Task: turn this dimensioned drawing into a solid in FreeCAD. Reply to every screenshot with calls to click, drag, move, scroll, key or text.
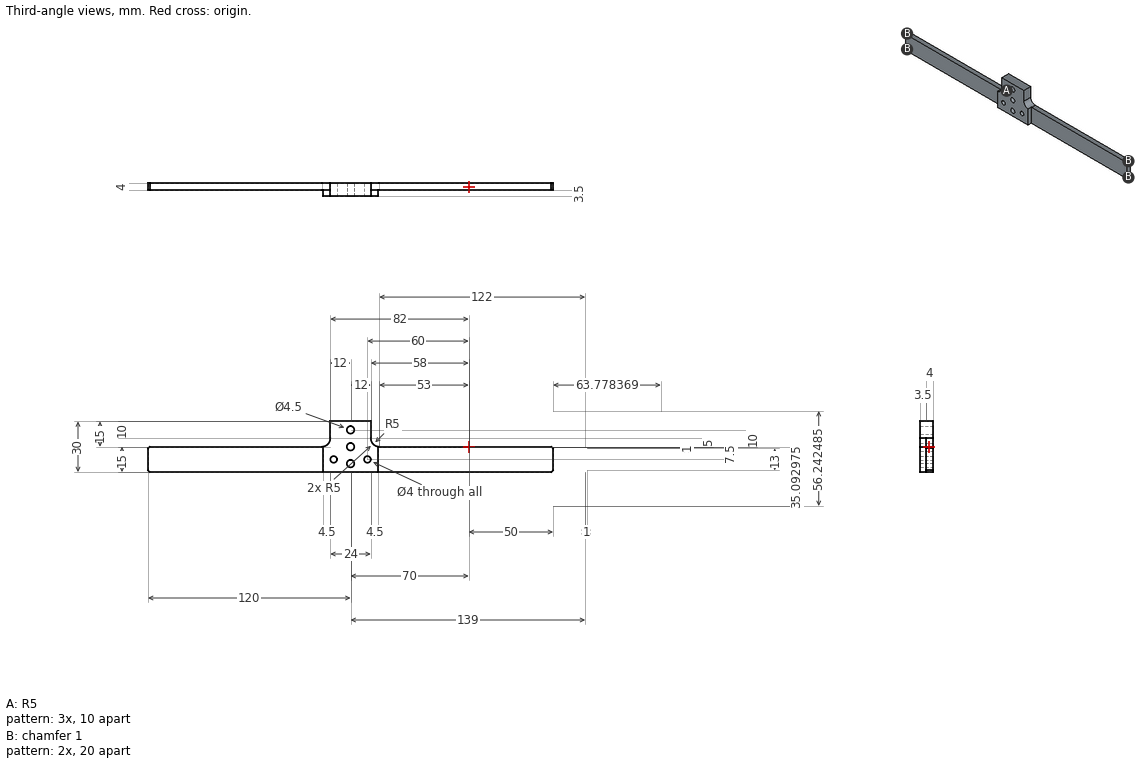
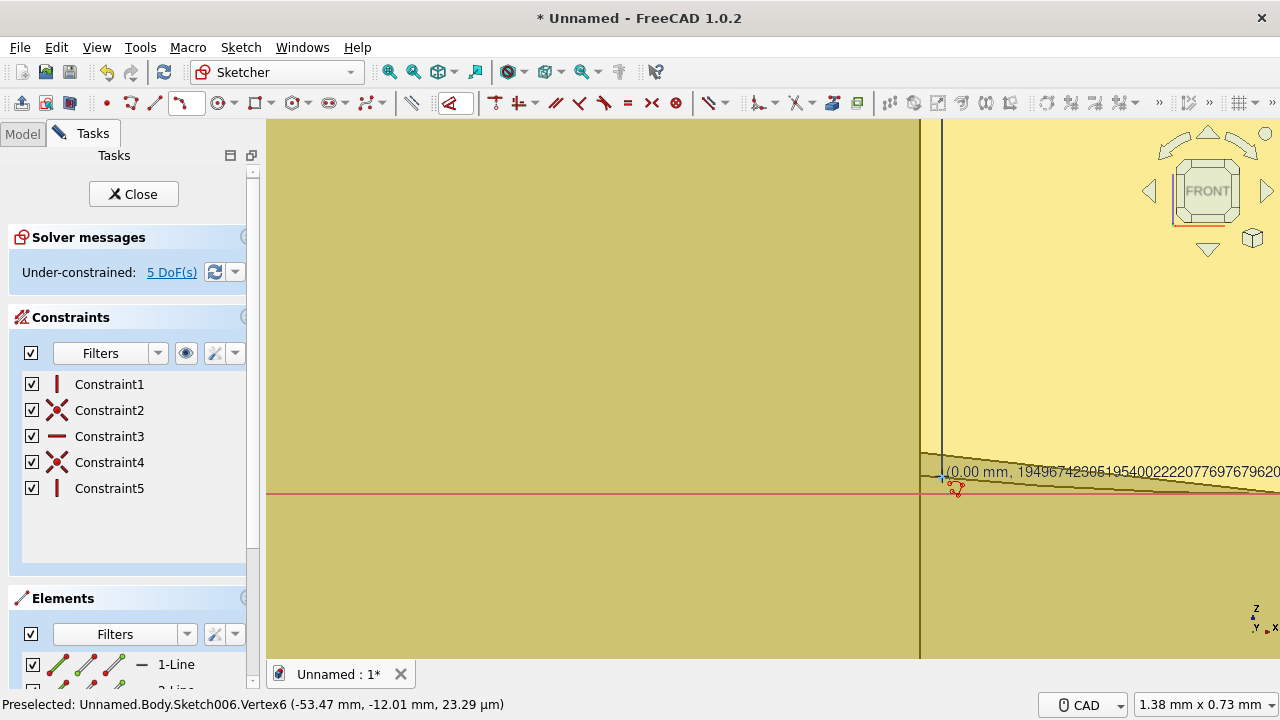
click(180, 104)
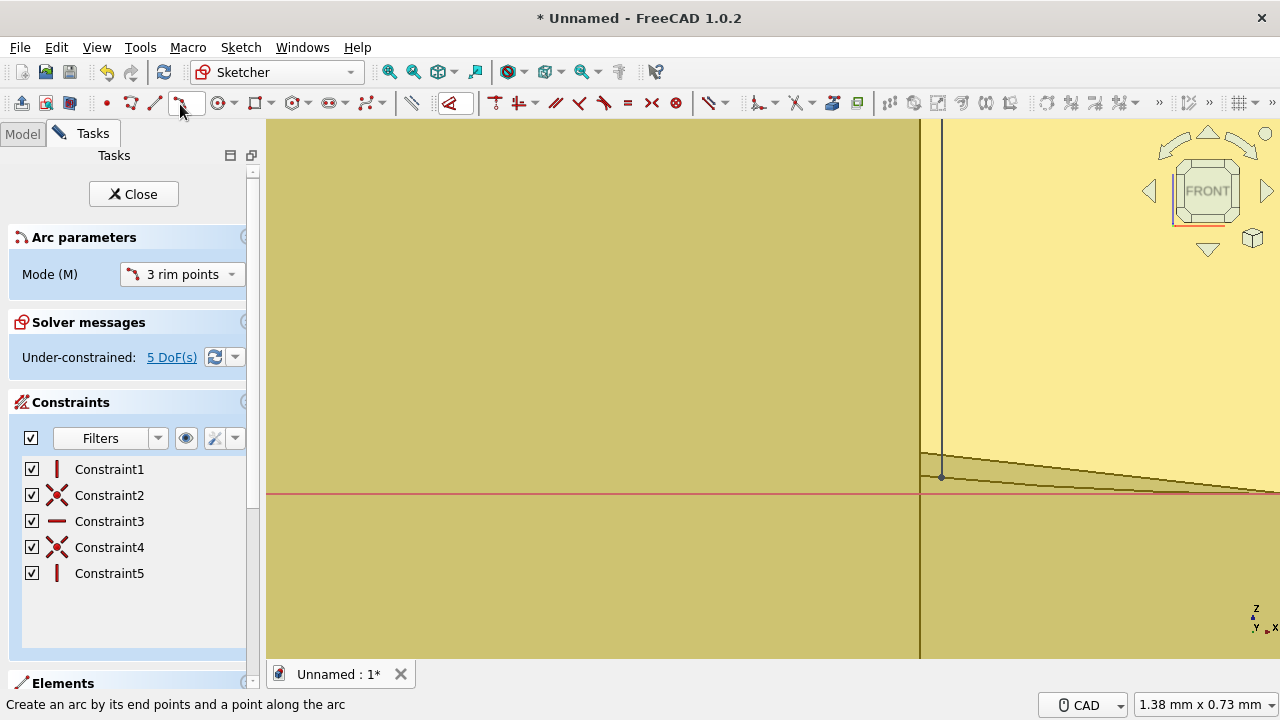
click(942, 477)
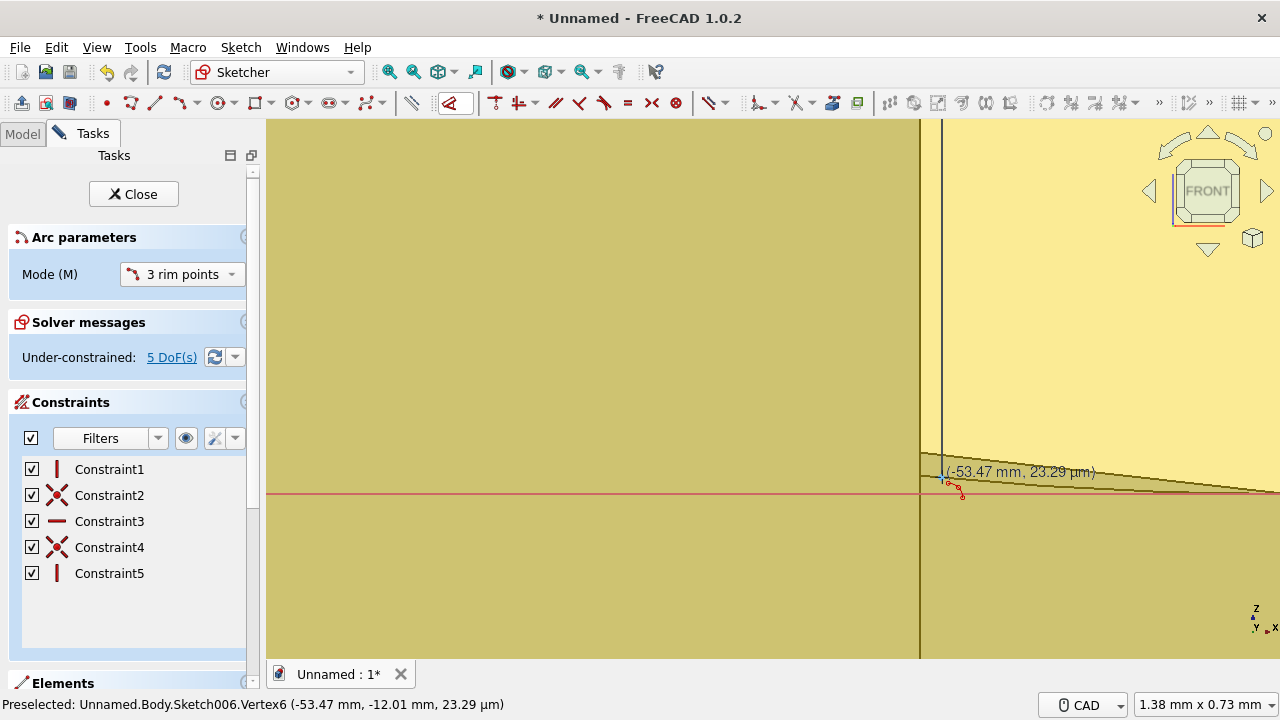
scroll(1040, 542, down, 18)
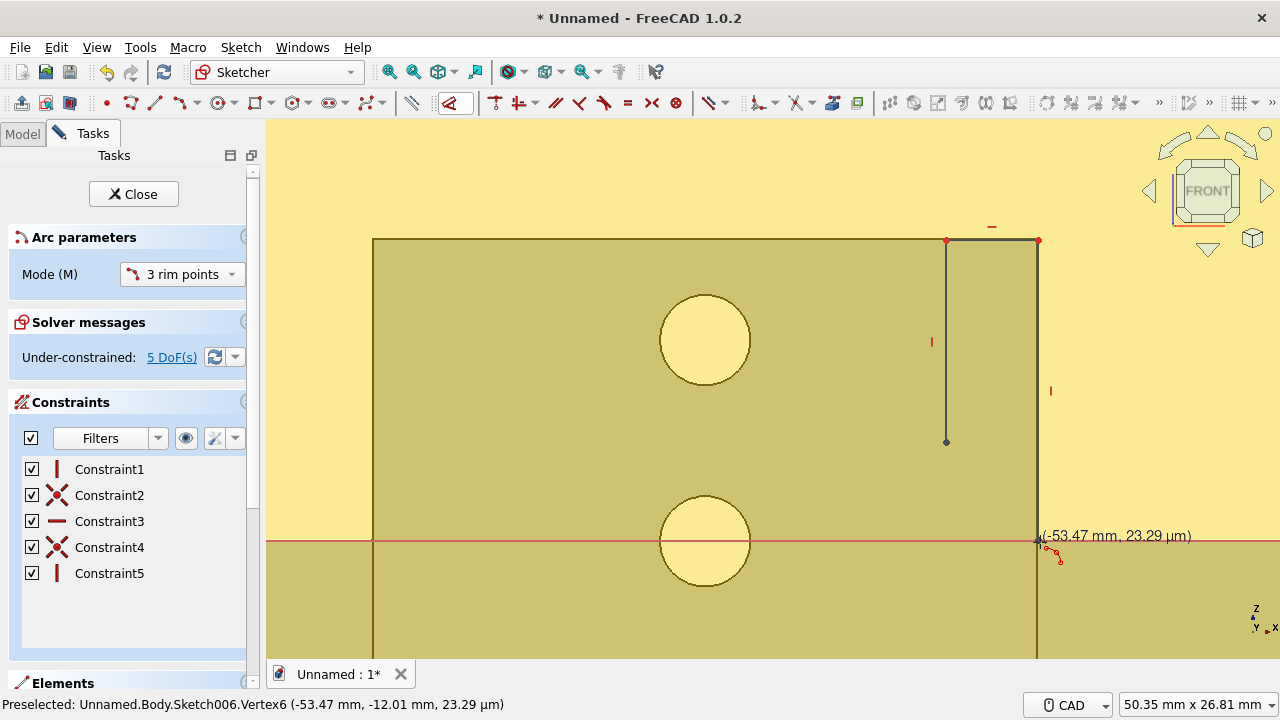
click(946, 442)
click(973, 508)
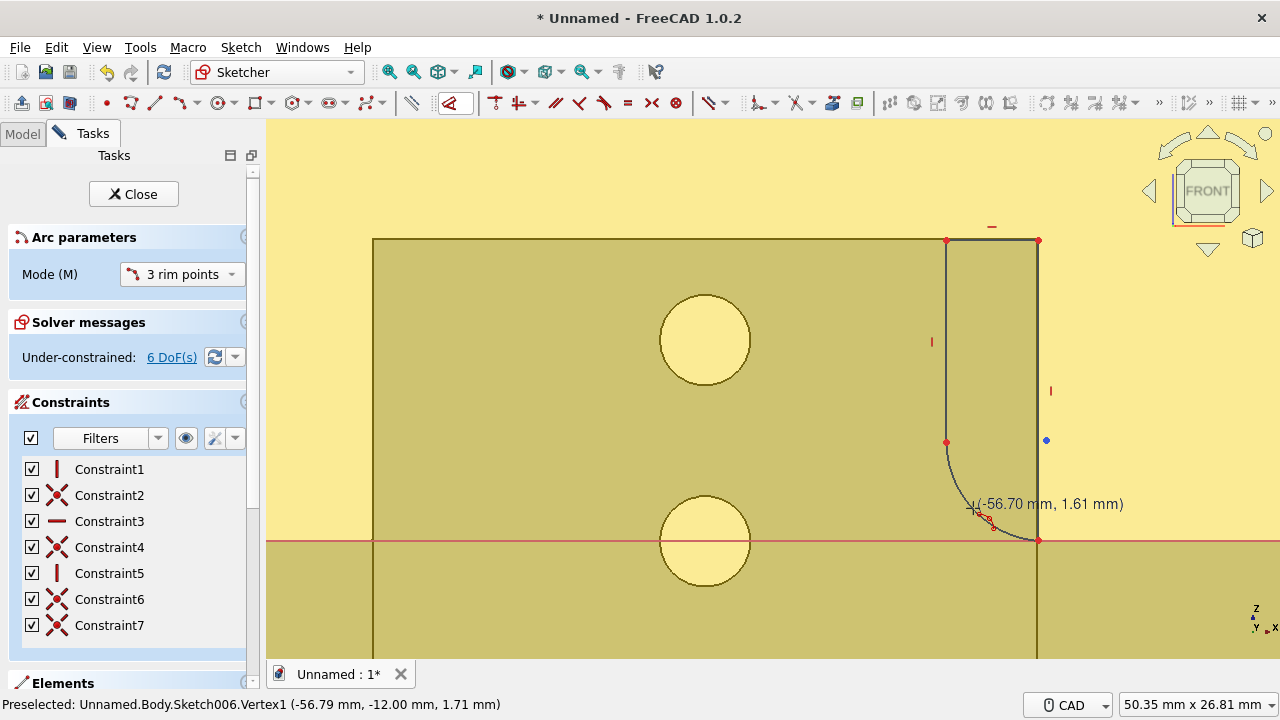
click(132, 104)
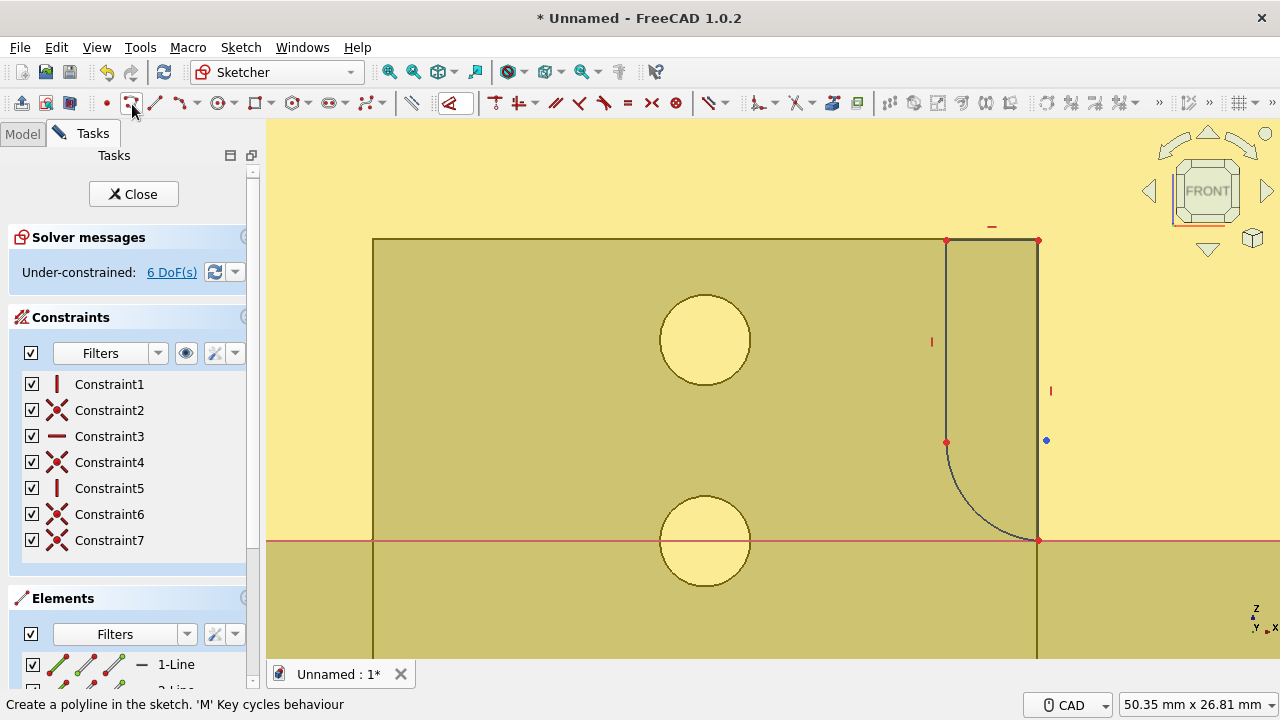
scroll(373, 541, up, 18)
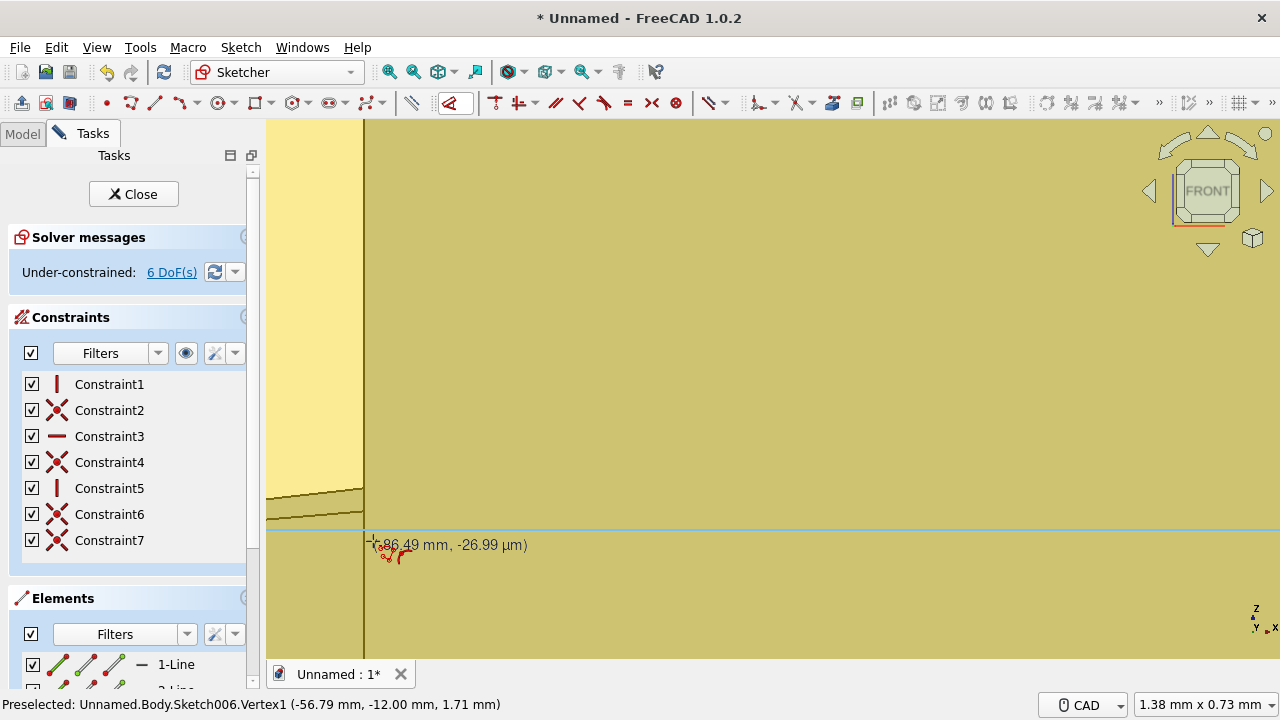
click(364, 511)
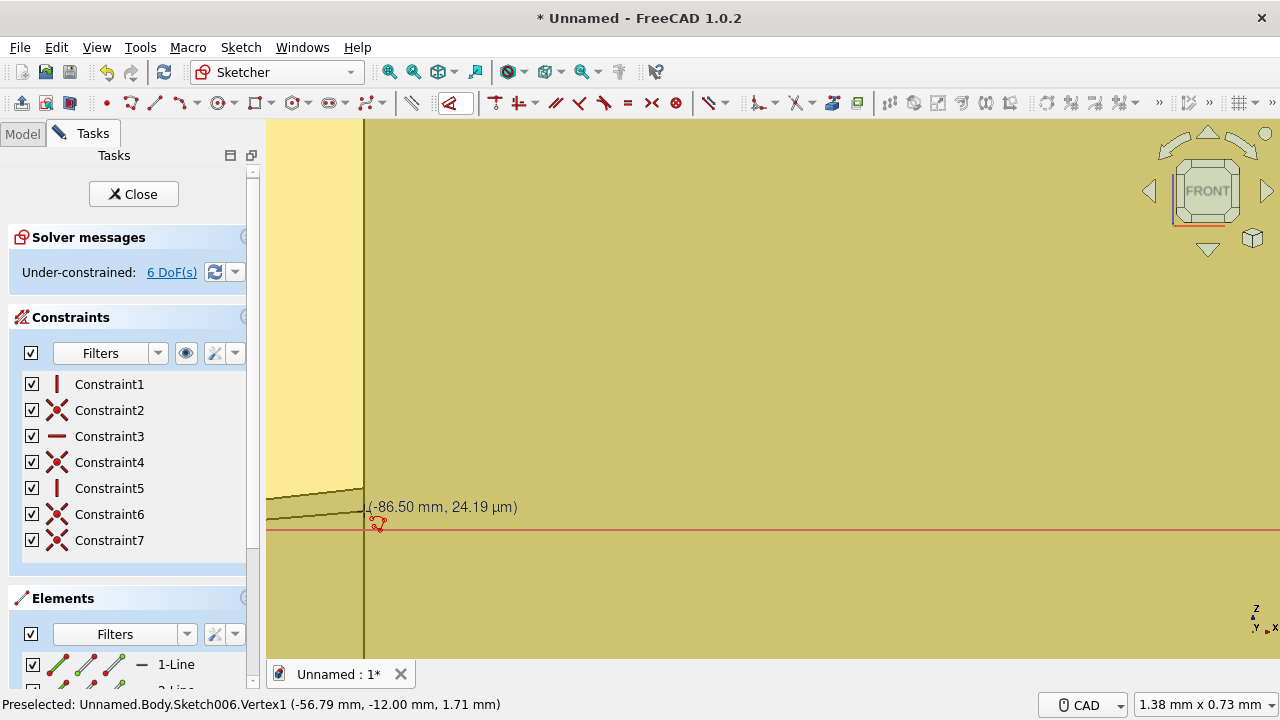
scroll(372, 541, down, 18)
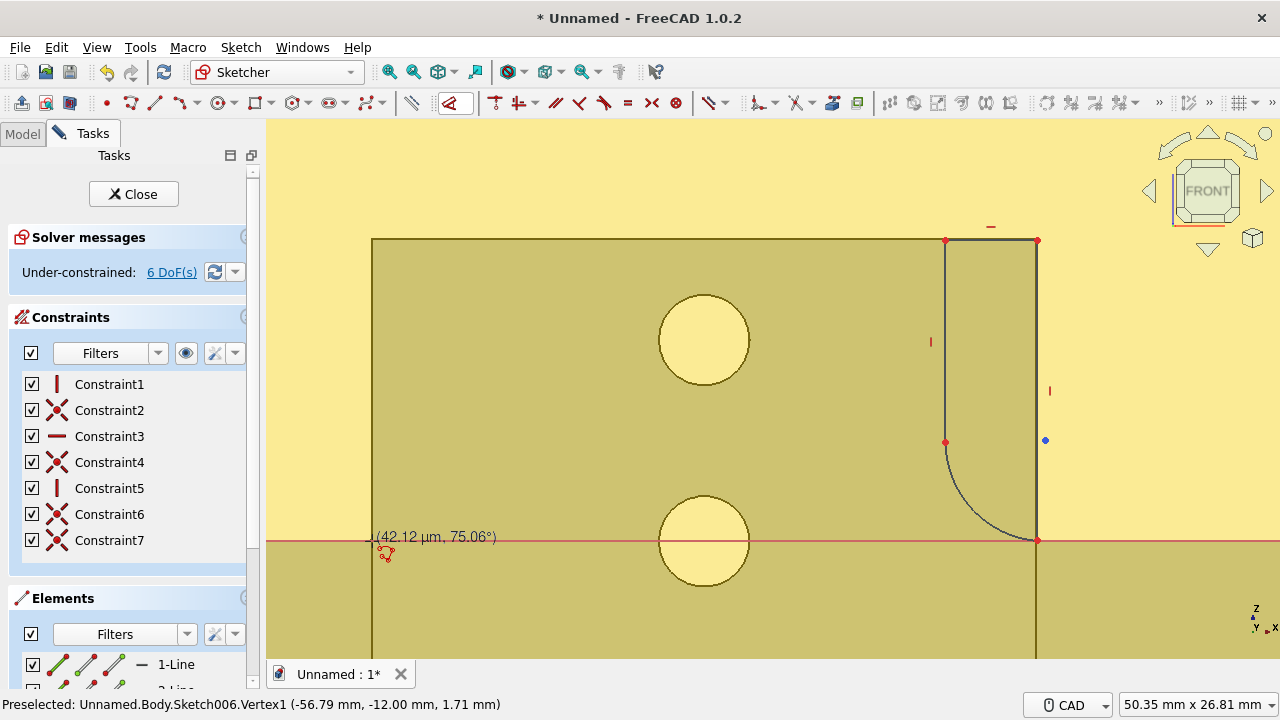
click(372, 239)
click(463, 239)
click(463, 441)
right_click(463, 441)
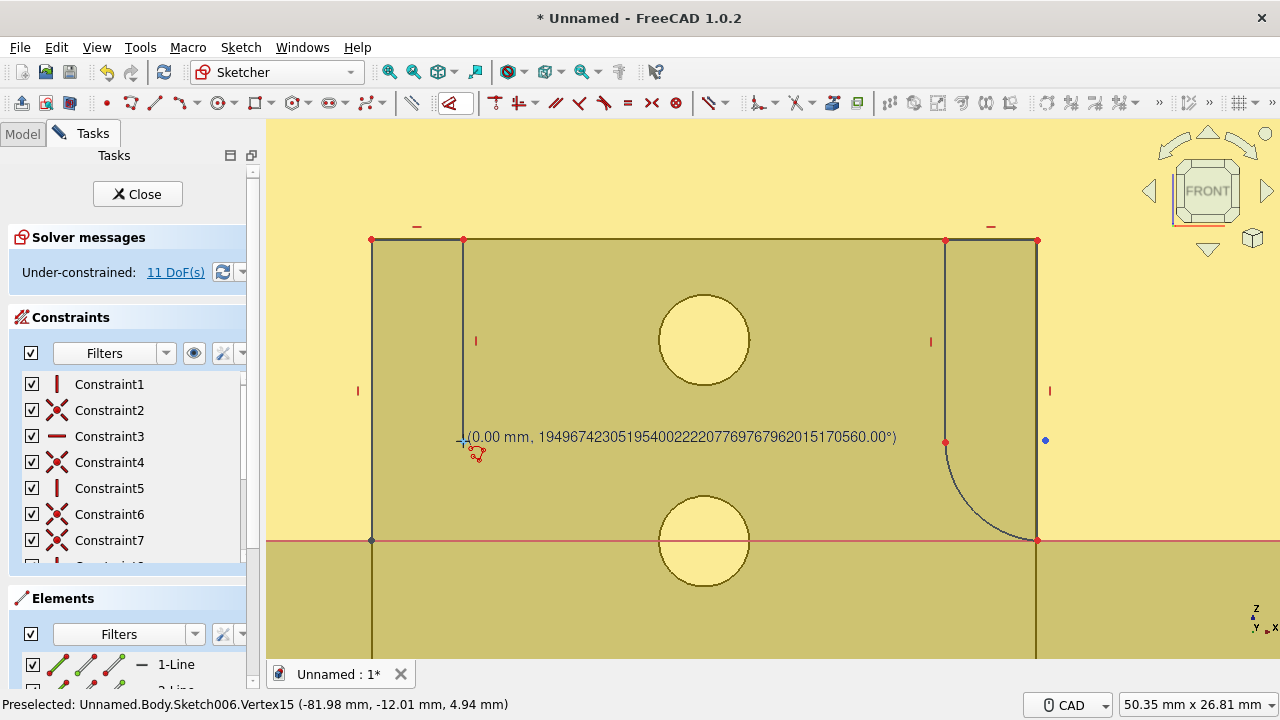
click(180, 104)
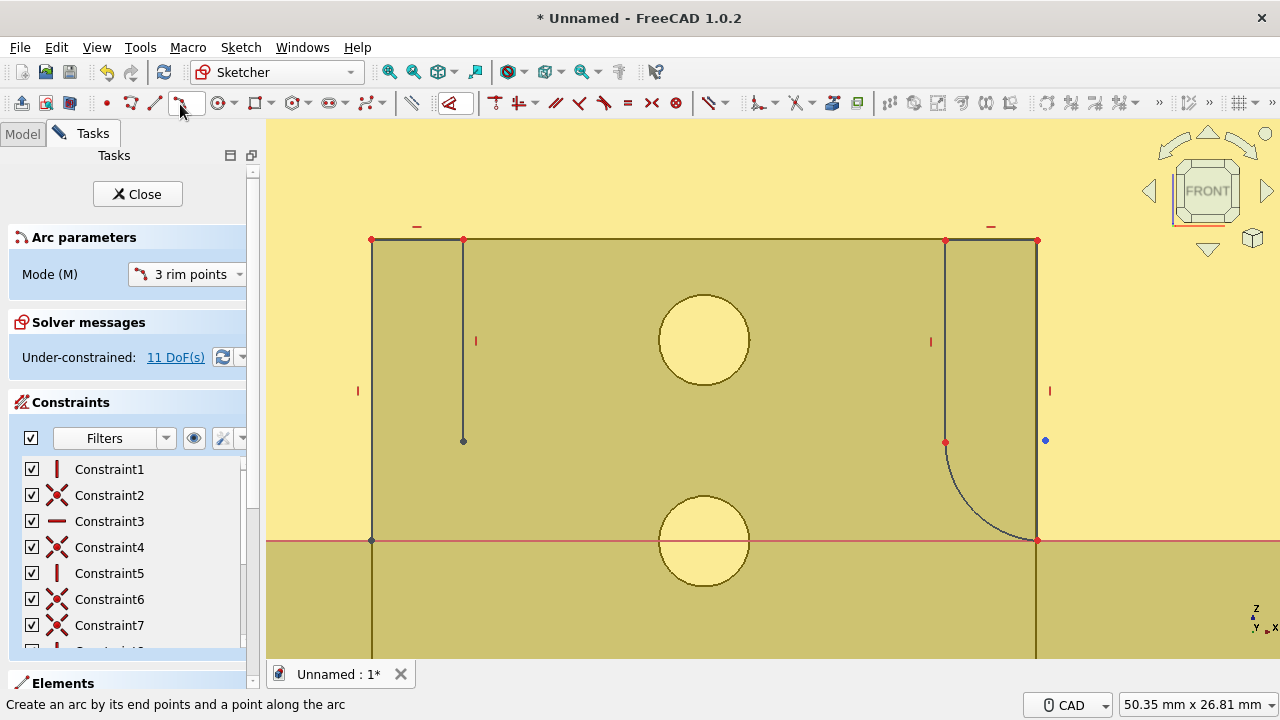
click(463, 442)